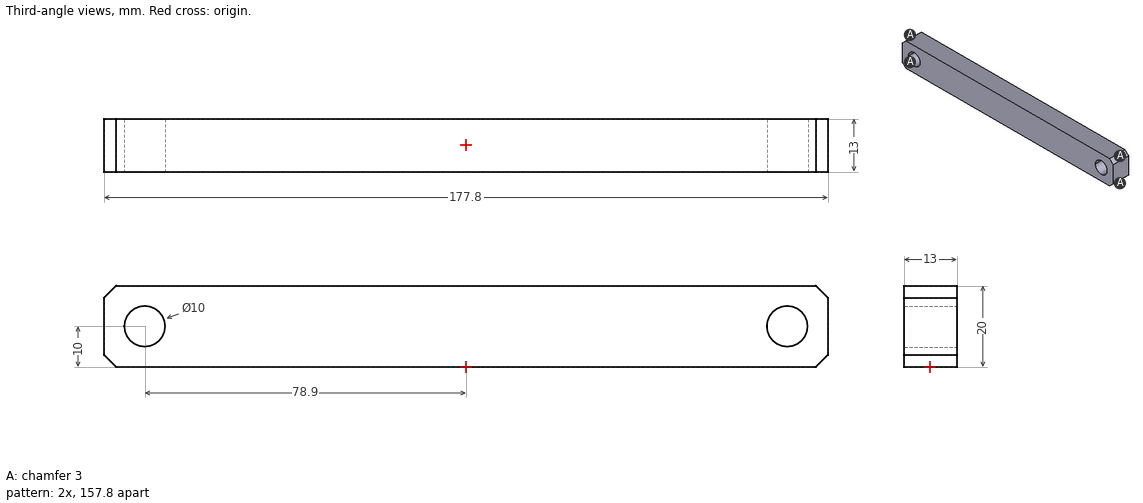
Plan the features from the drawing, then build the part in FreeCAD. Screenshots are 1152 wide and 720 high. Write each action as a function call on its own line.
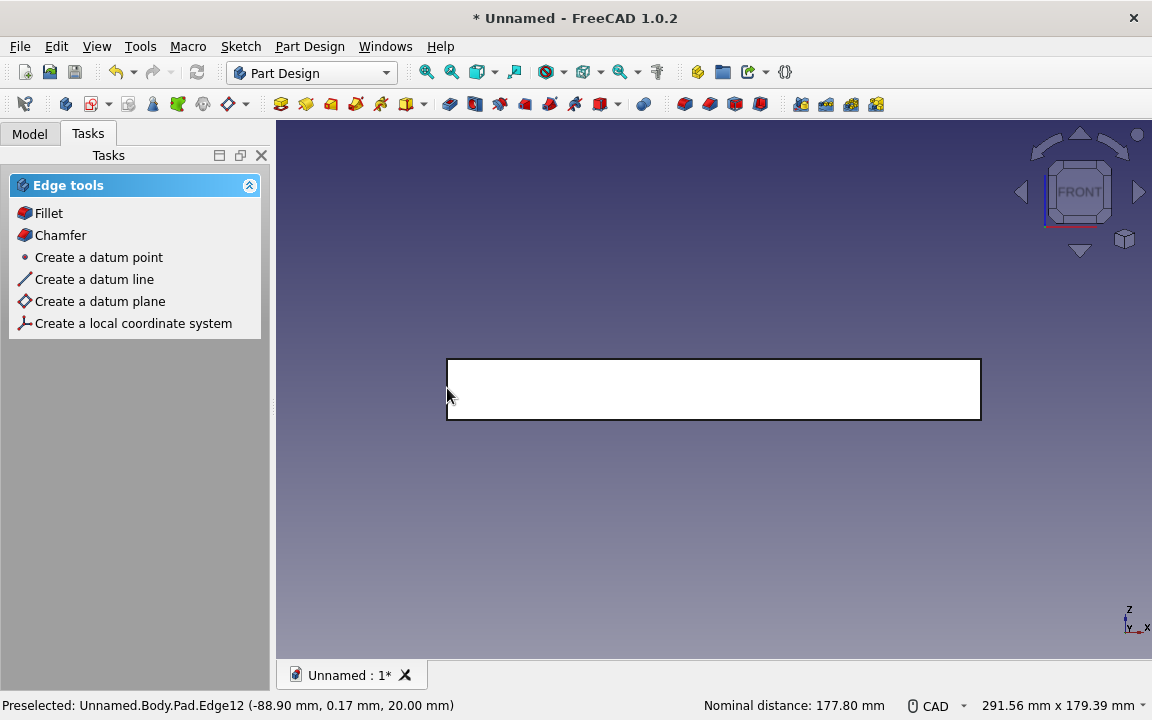
key(3)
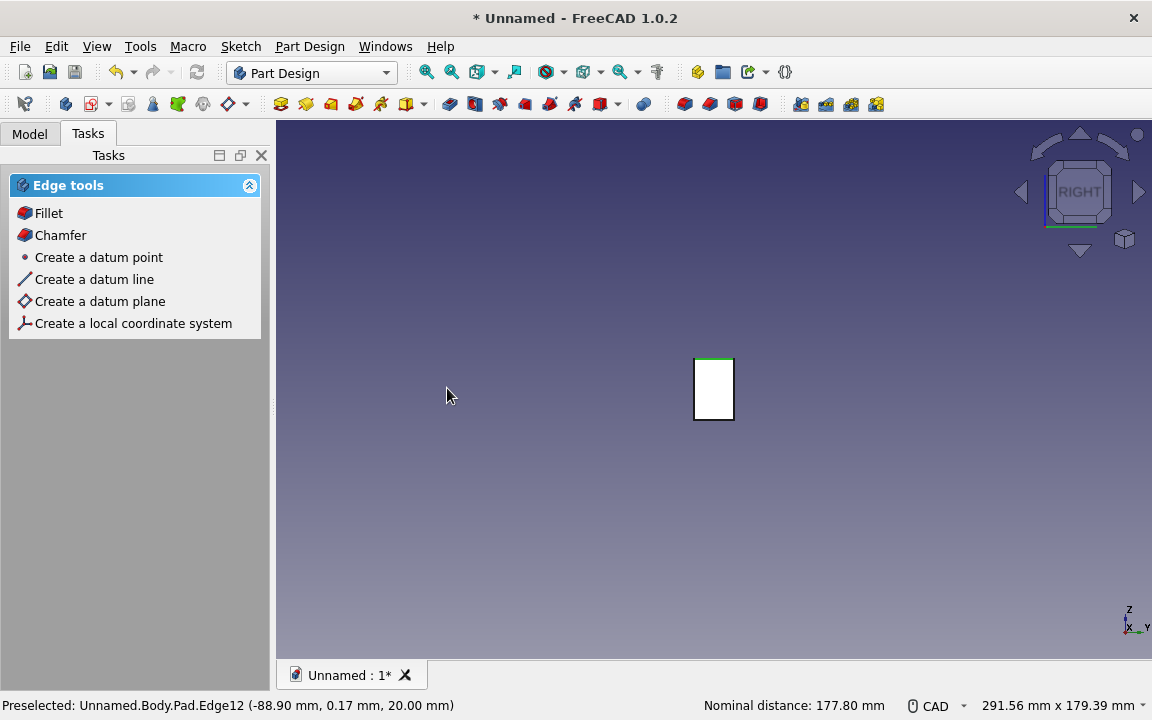
click(427, 72)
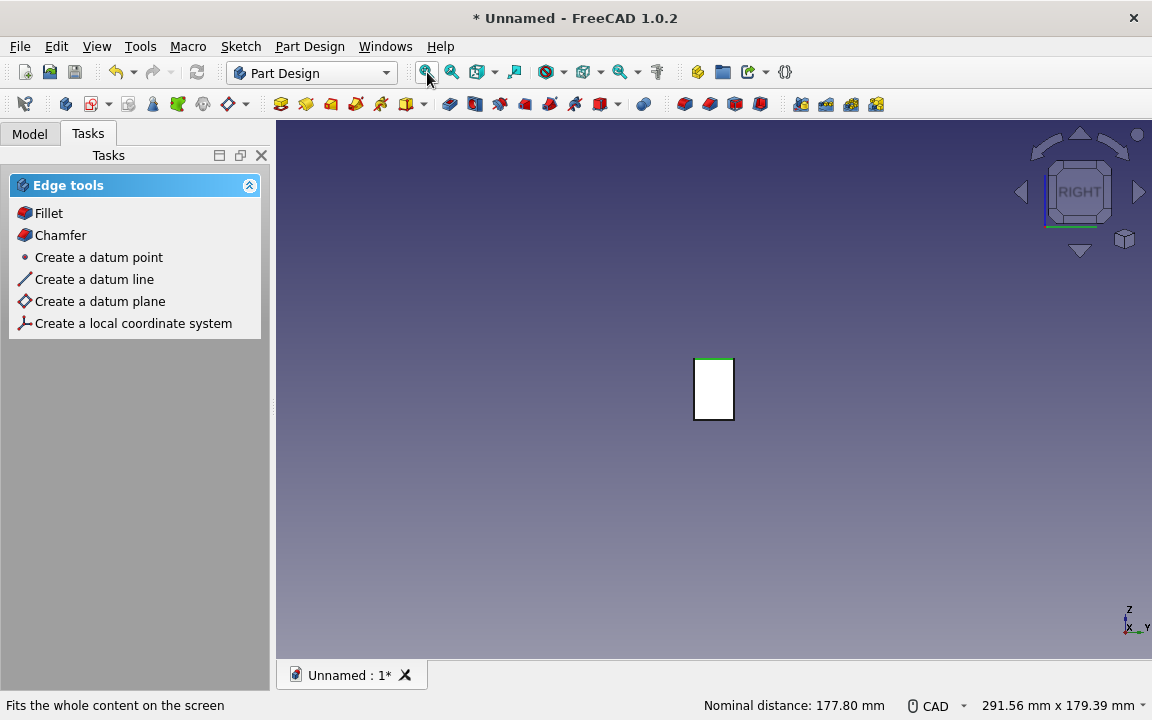
click(714, 419, ctrl)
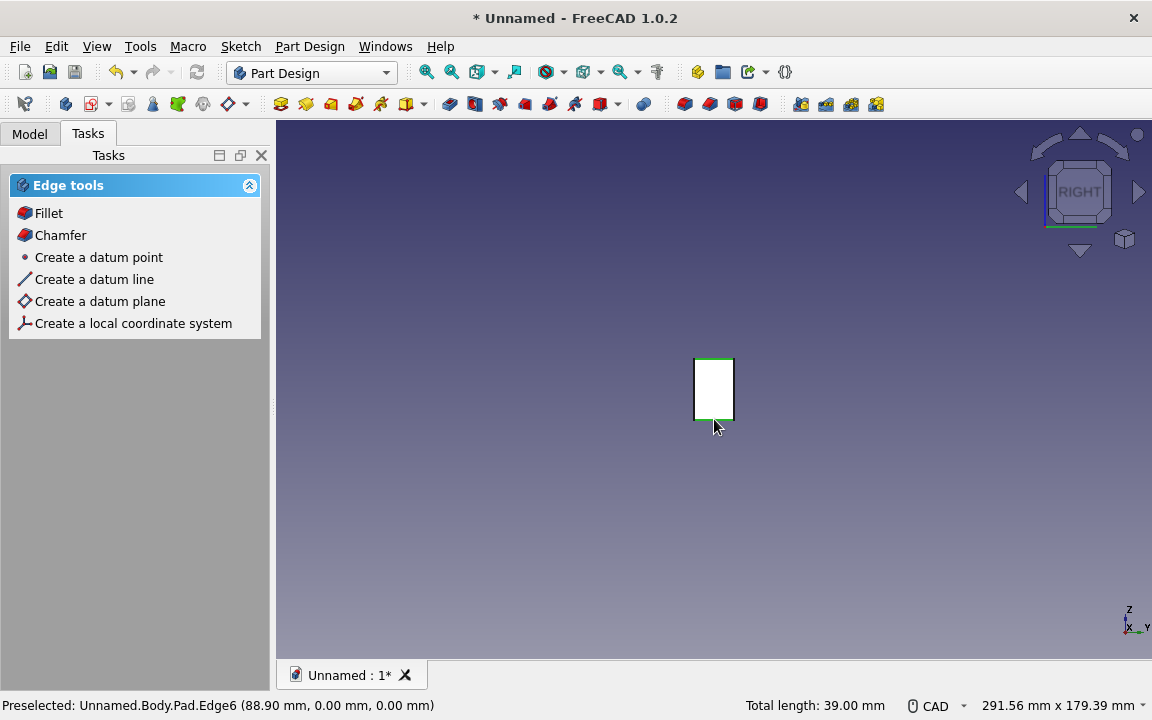
key(5)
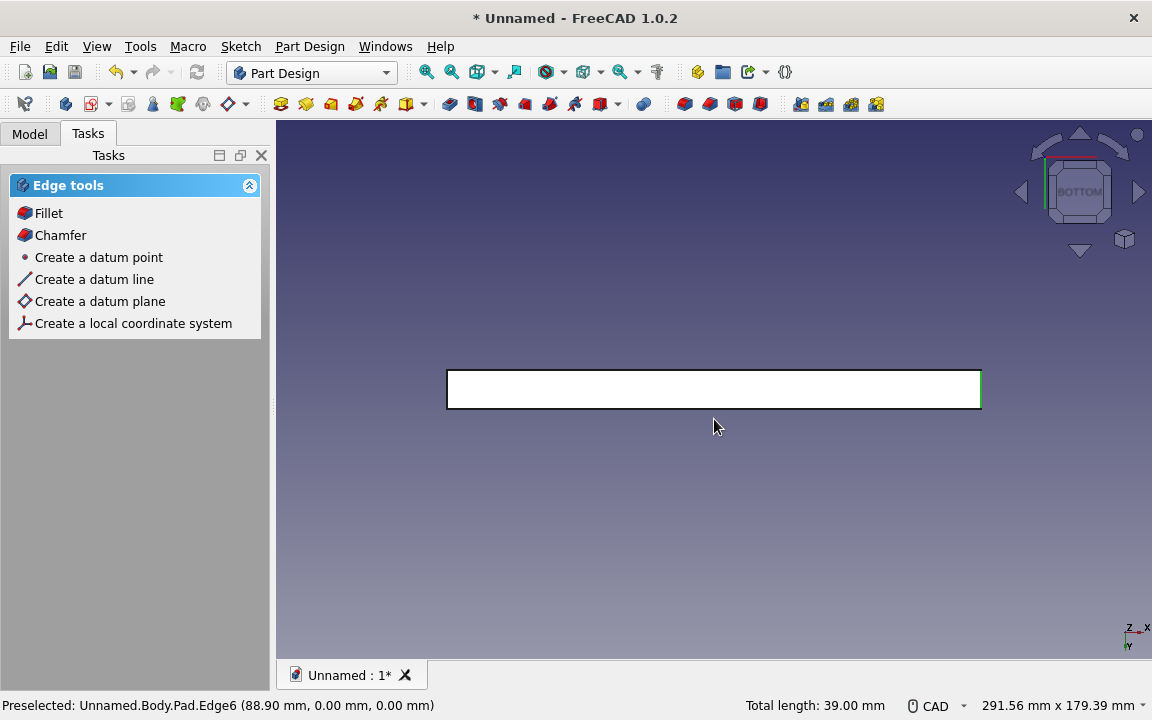
click(447, 388, ctrl)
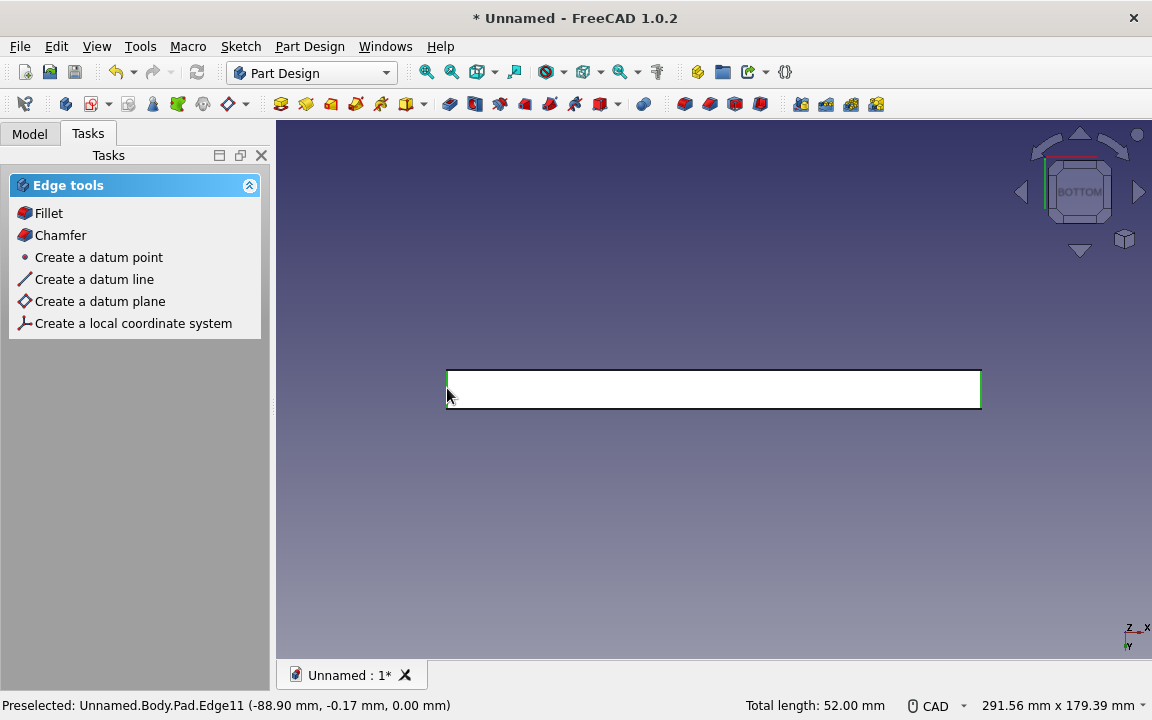
click(710, 104)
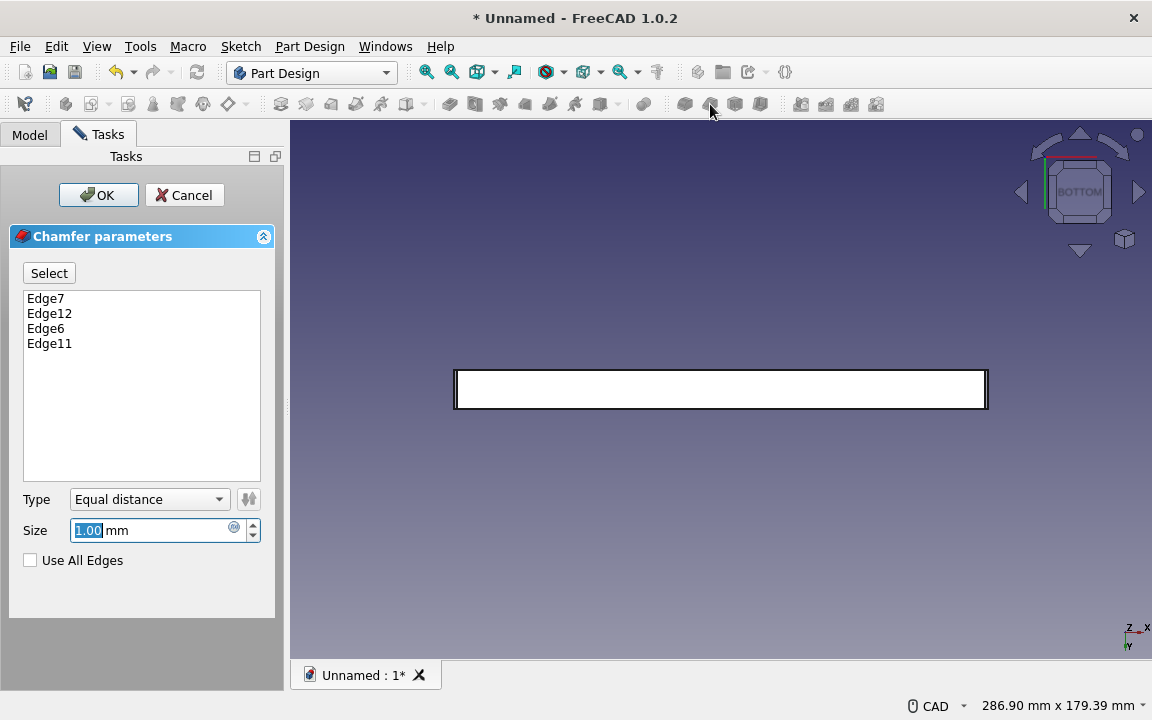
text(3)
key(Tab)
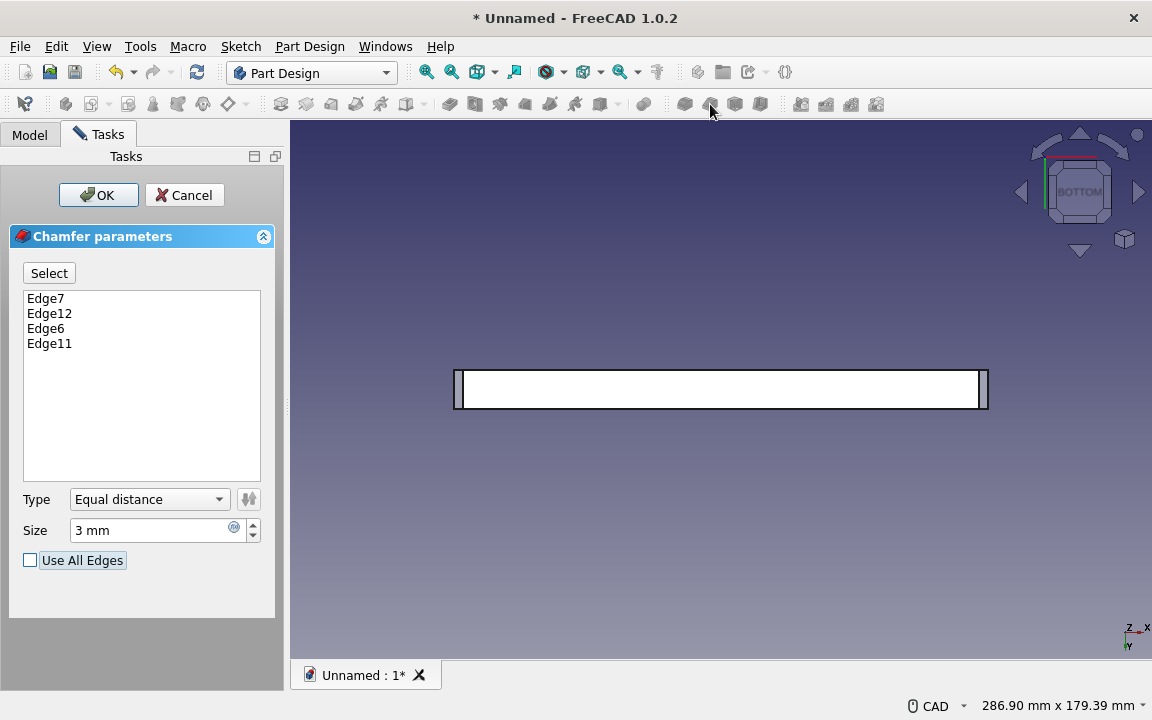
click(99, 195)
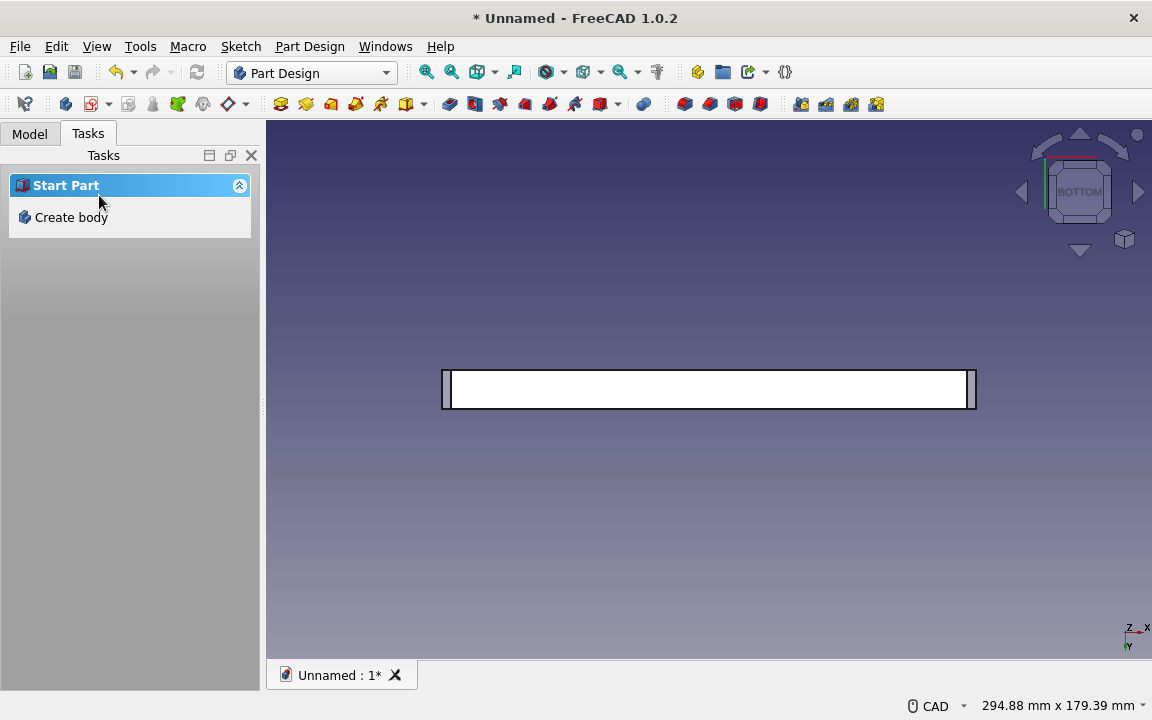
key(4)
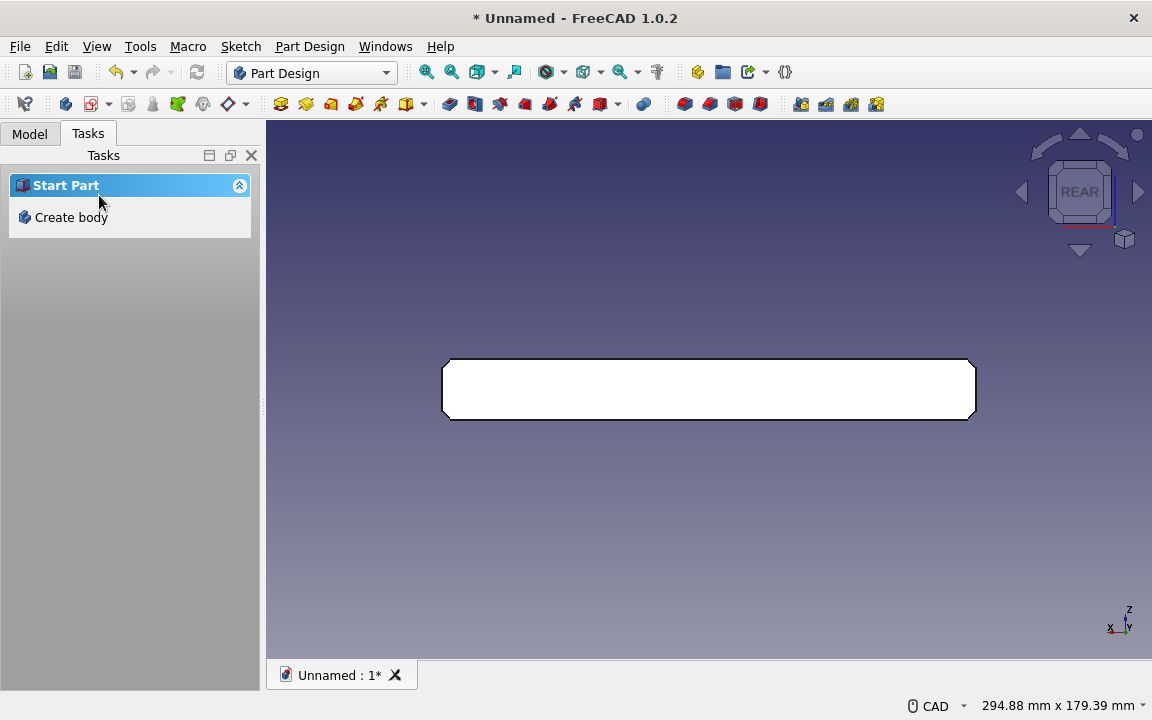
click(480, 389)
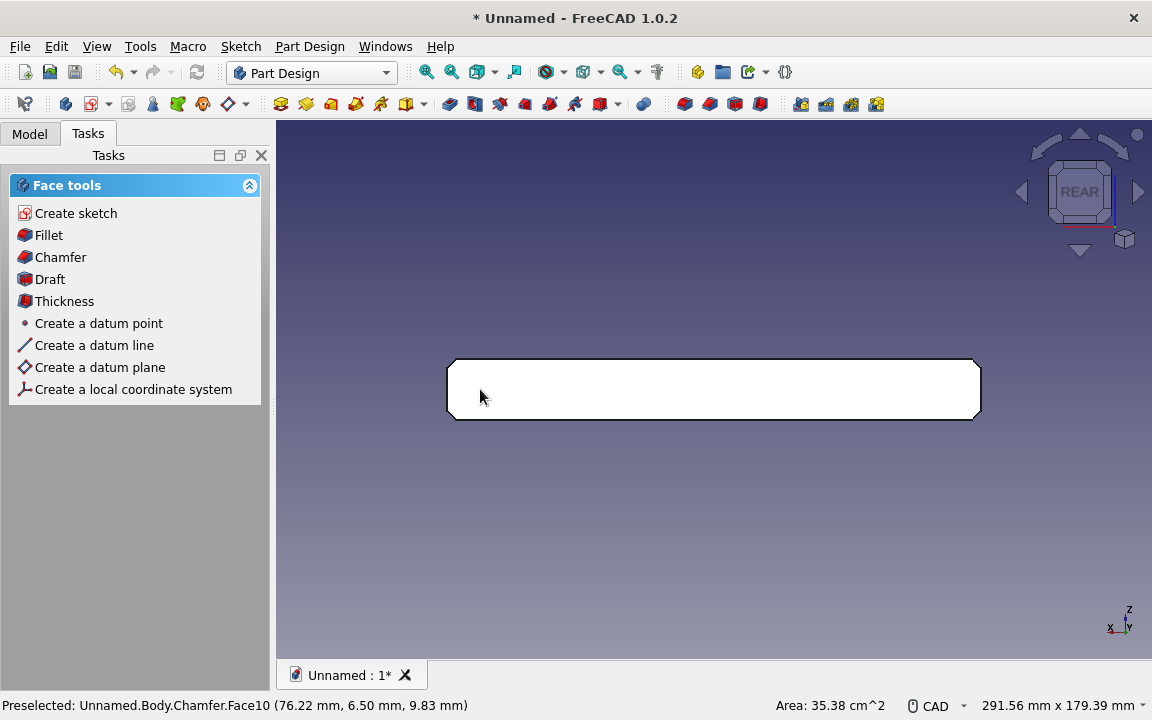
click(90, 104)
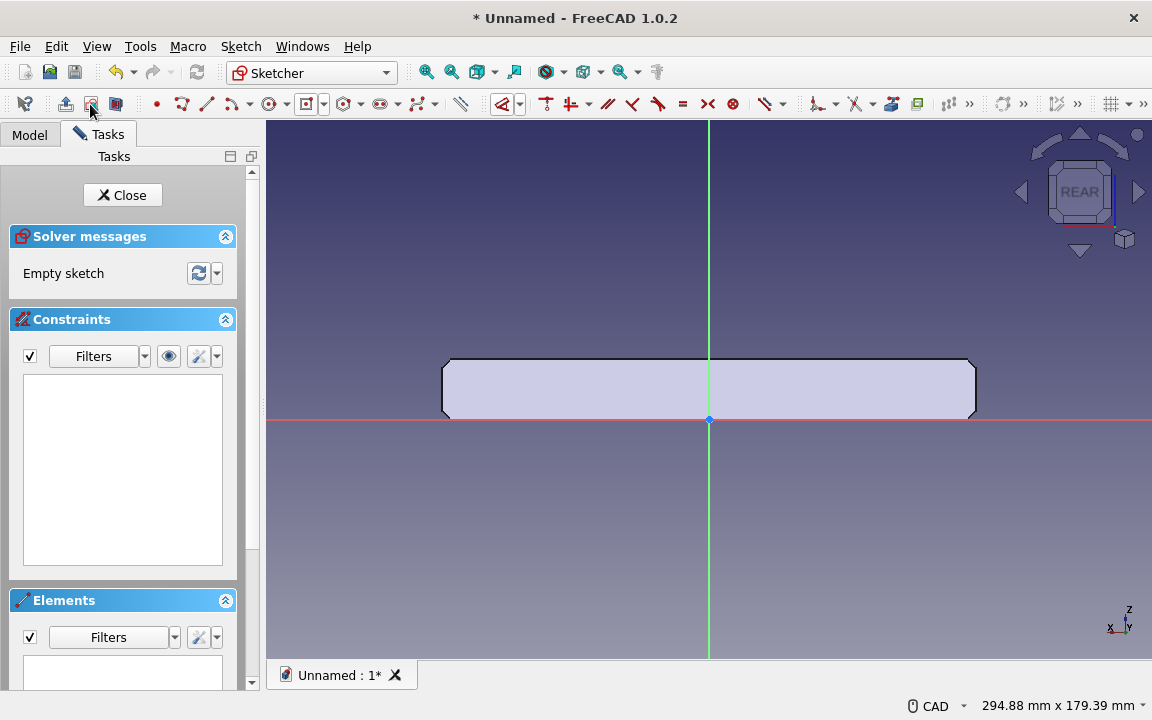
scroll(977, 390, up, 12)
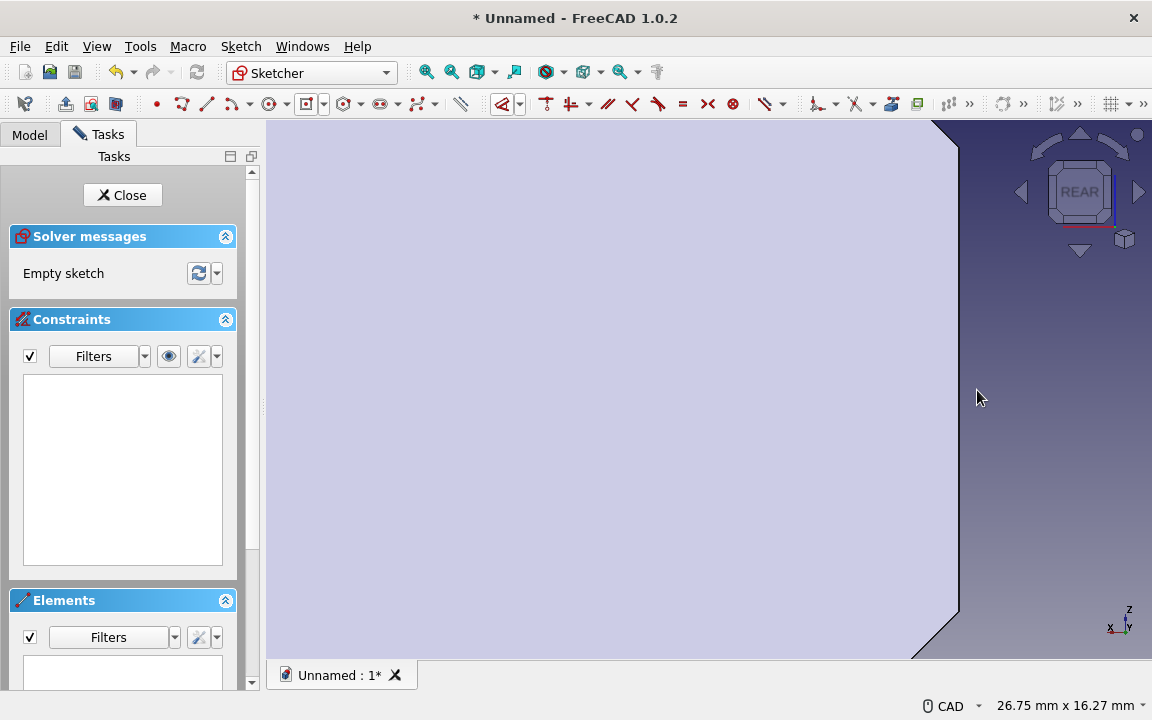
click(268, 104)